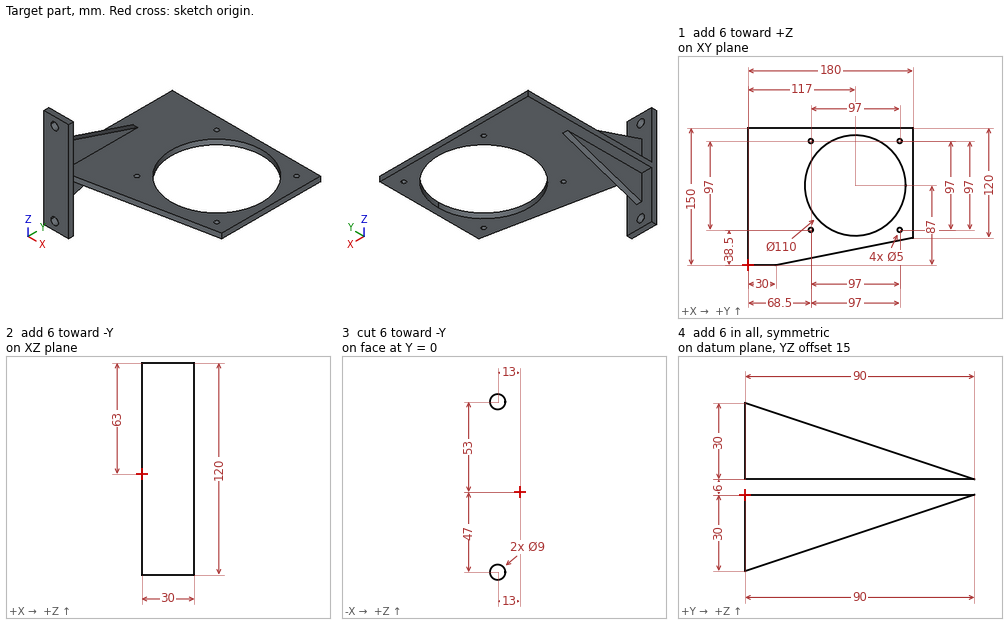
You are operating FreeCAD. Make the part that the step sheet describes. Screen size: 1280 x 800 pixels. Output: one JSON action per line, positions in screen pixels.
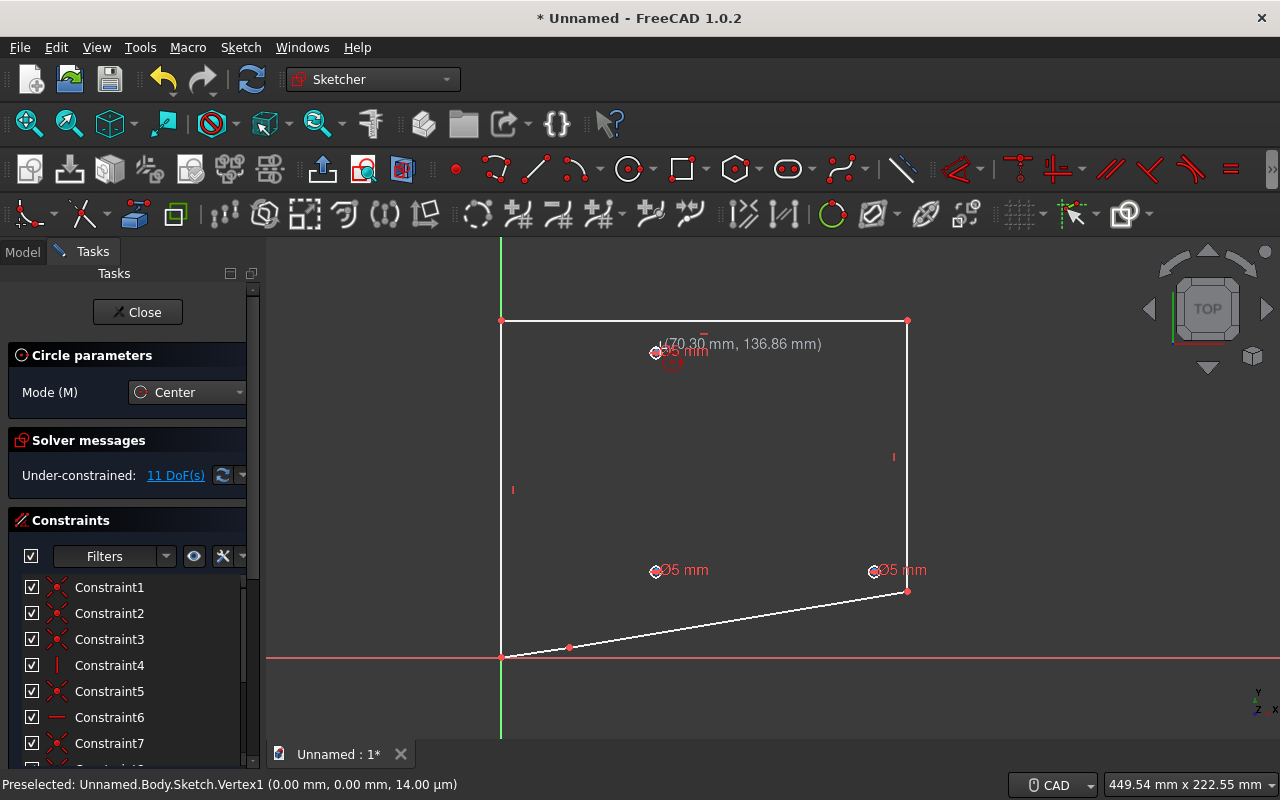
{"action": "left_click", "coordinate": [765, 461]}
{"action": "mouse_move", "coordinate": [853, 374]}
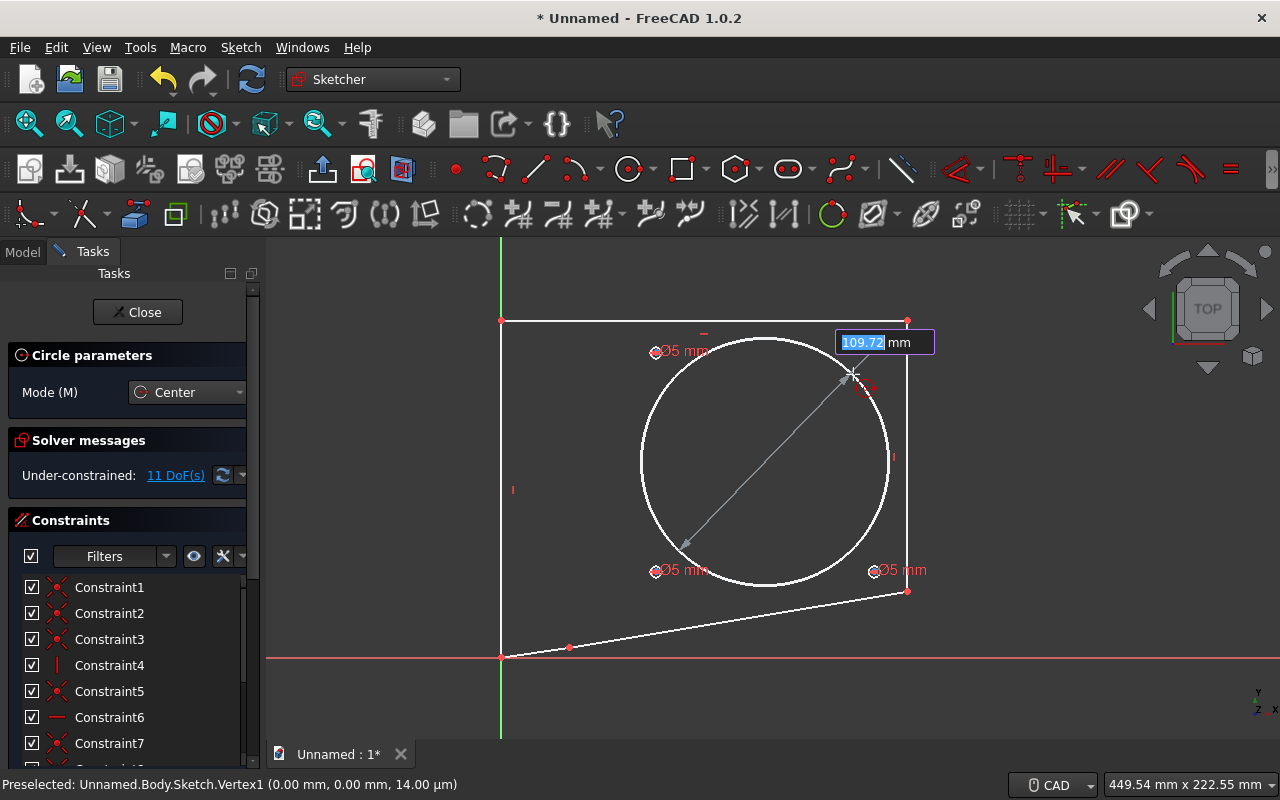
{"action": "type", "text": "110"}
{"action": "key", "text": "Return"}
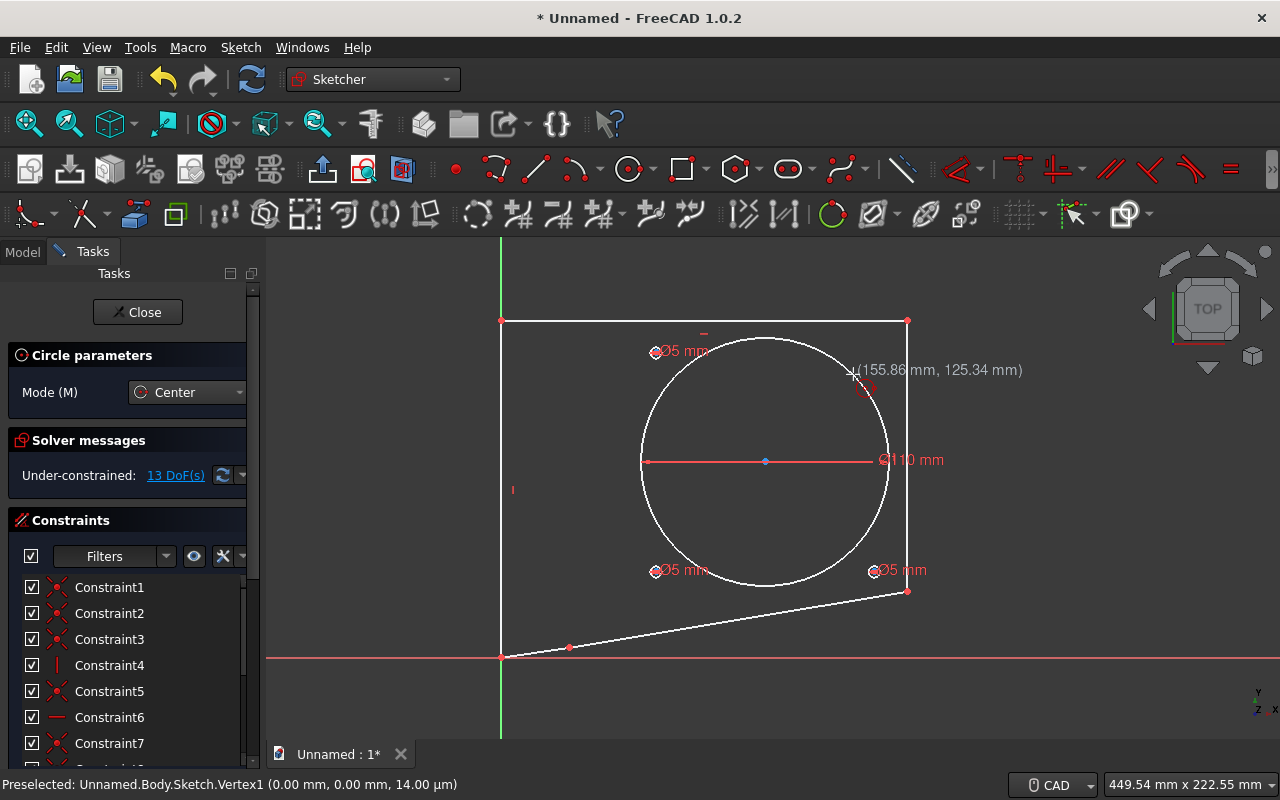
{"action": "scroll", "coordinate": [875, 352], "scroll_direction": "up", "scroll_amount": 7}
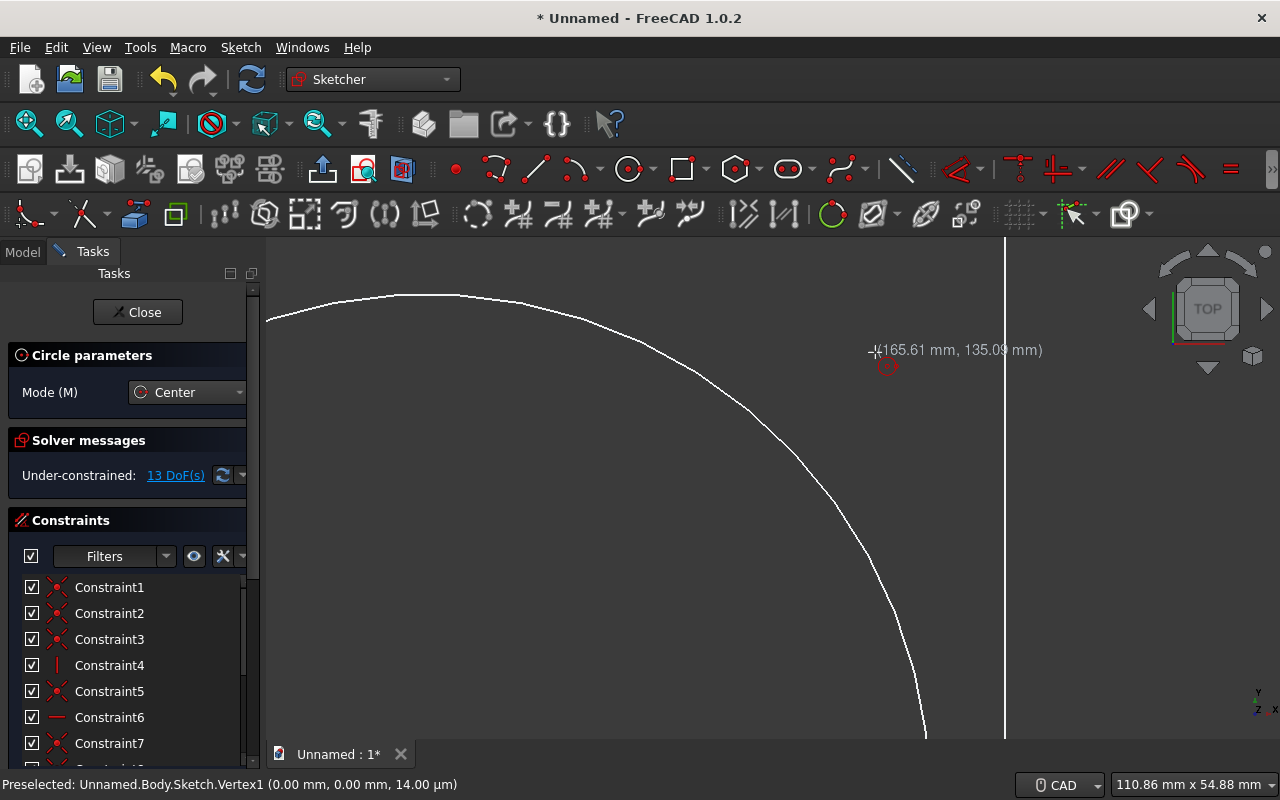
{"action": "scroll", "coordinate": [876, 352], "scroll_direction": "down", "scroll_amount": 7}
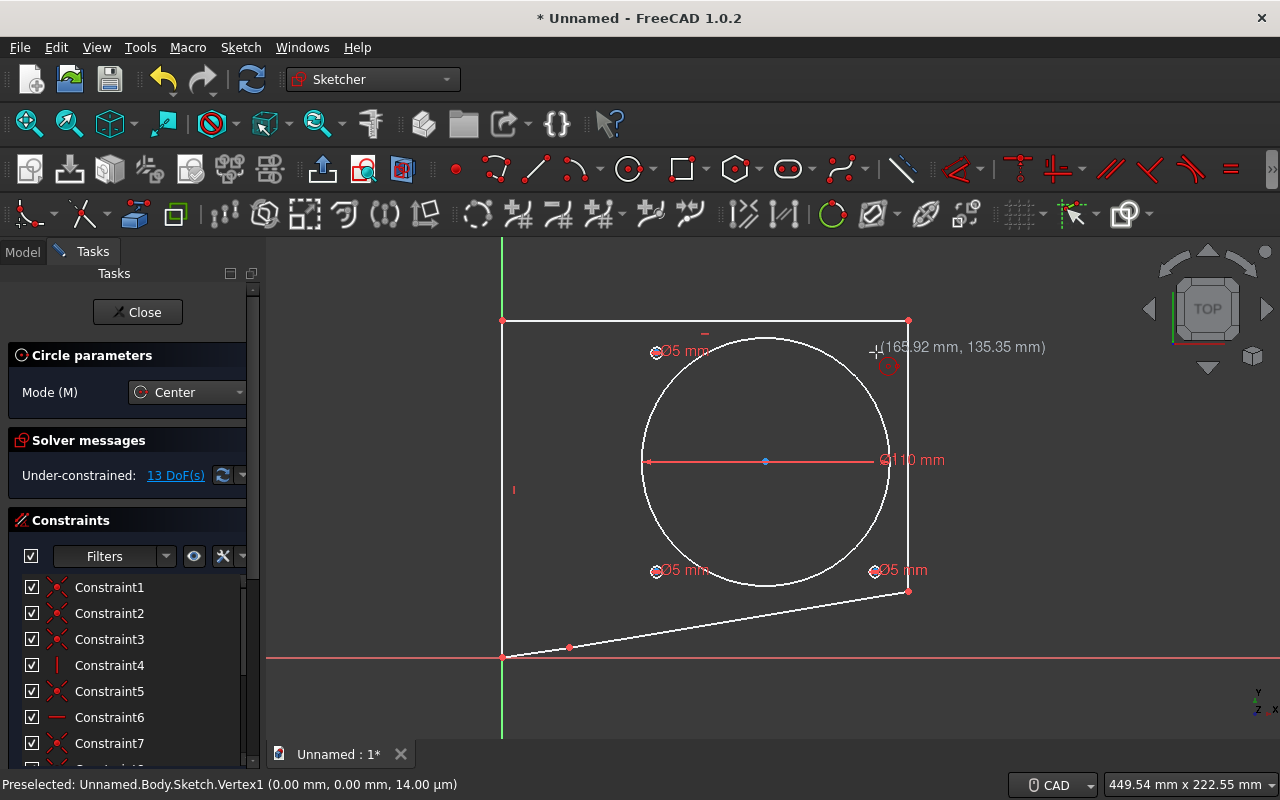
{"action": "left_click", "coordinate": [875, 352]}
{"action": "mouse_move", "coordinate": [879, 348]}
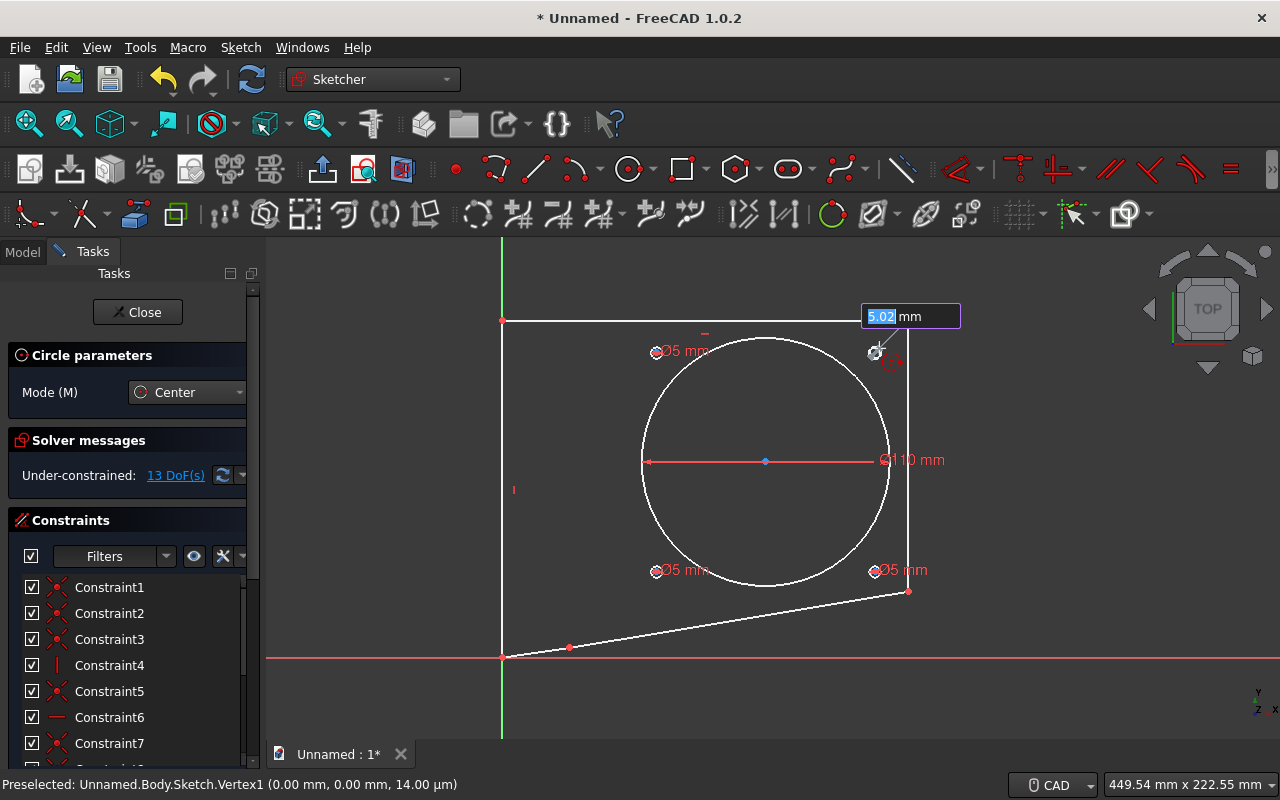
{"action": "type", "text": "5"}
{"action": "key", "text": "Return"}
{"action": "key", "text": "Escape"}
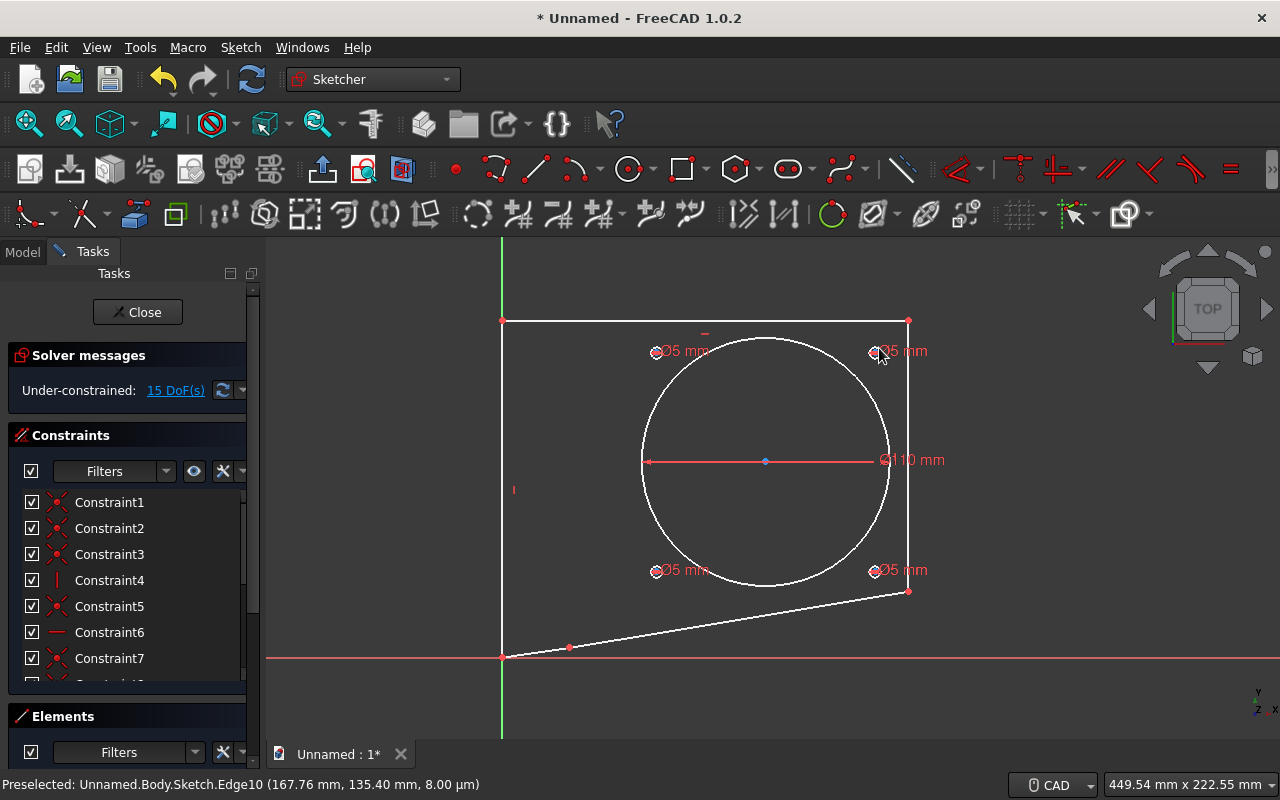
{"action": "left_click", "coordinate": [523, 655]}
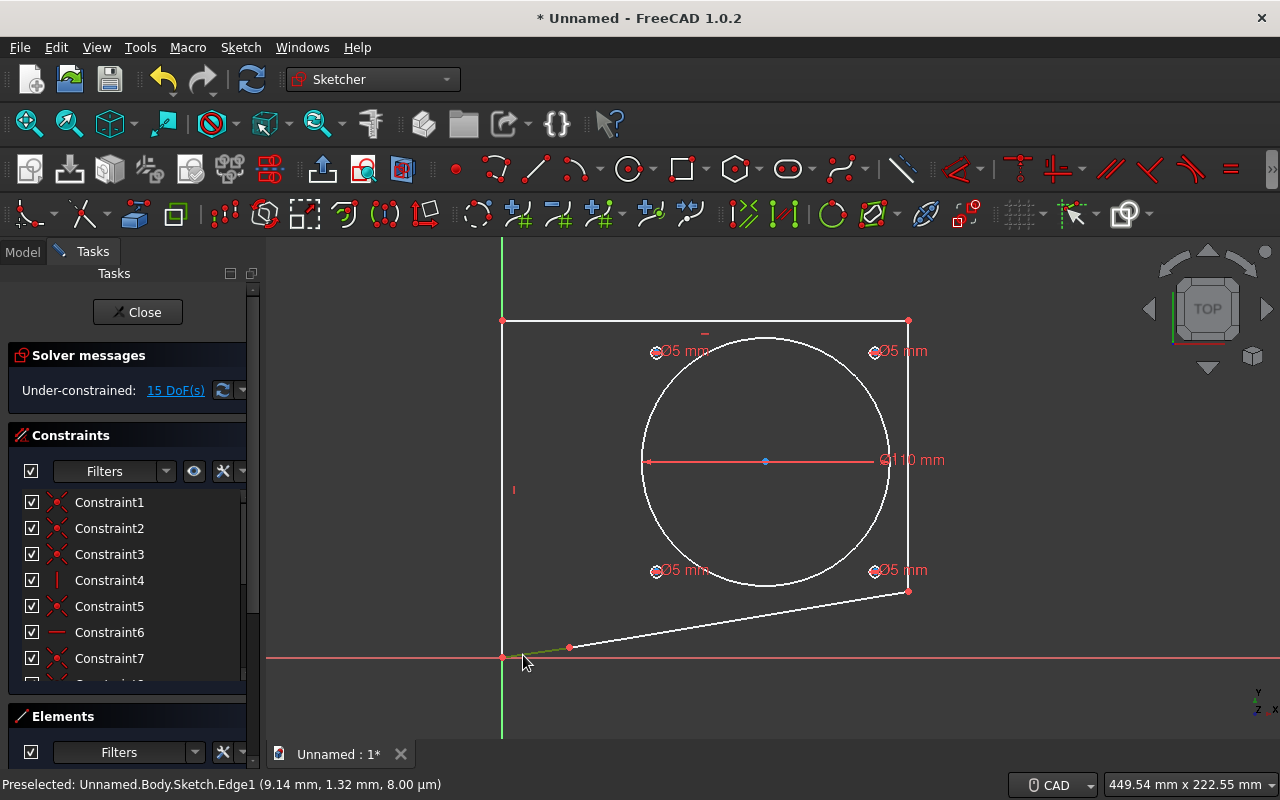
{"action": "key", "text": "h"}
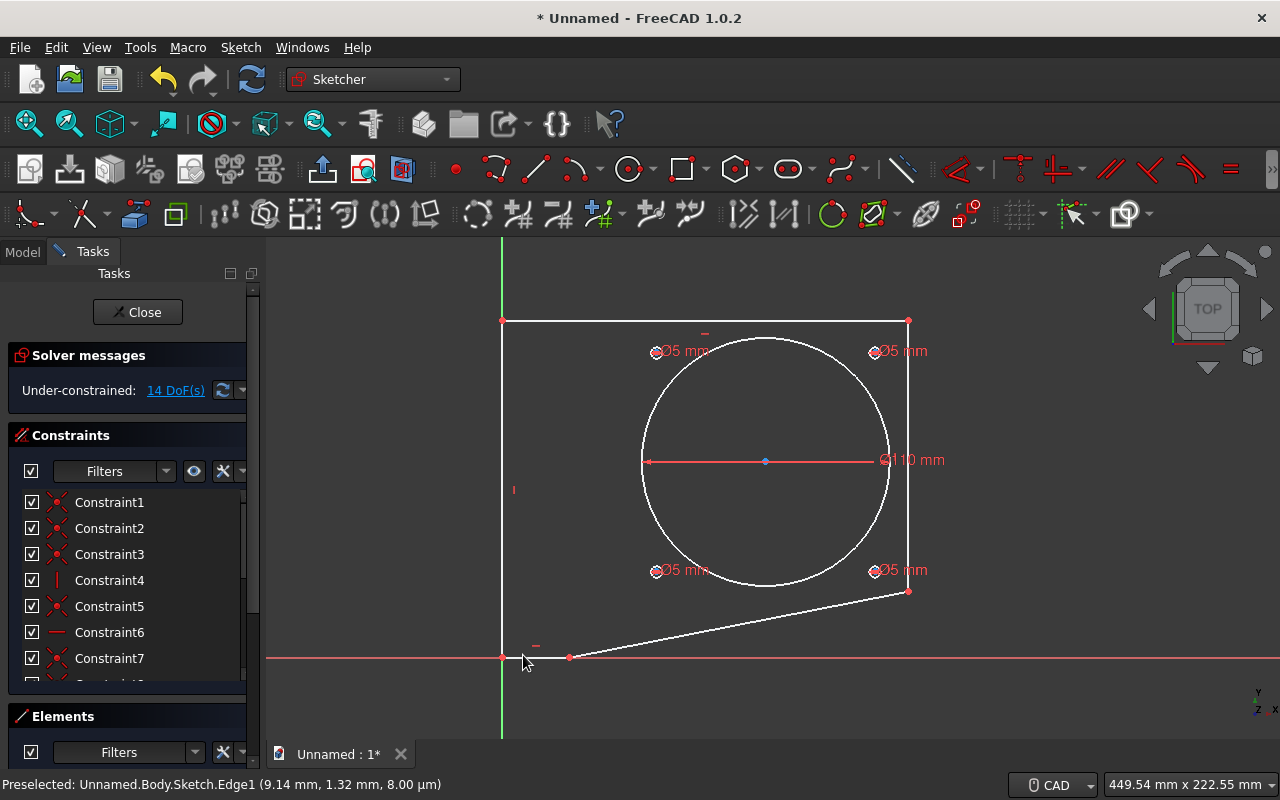
{"action": "left_click", "coordinate": [523, 658]}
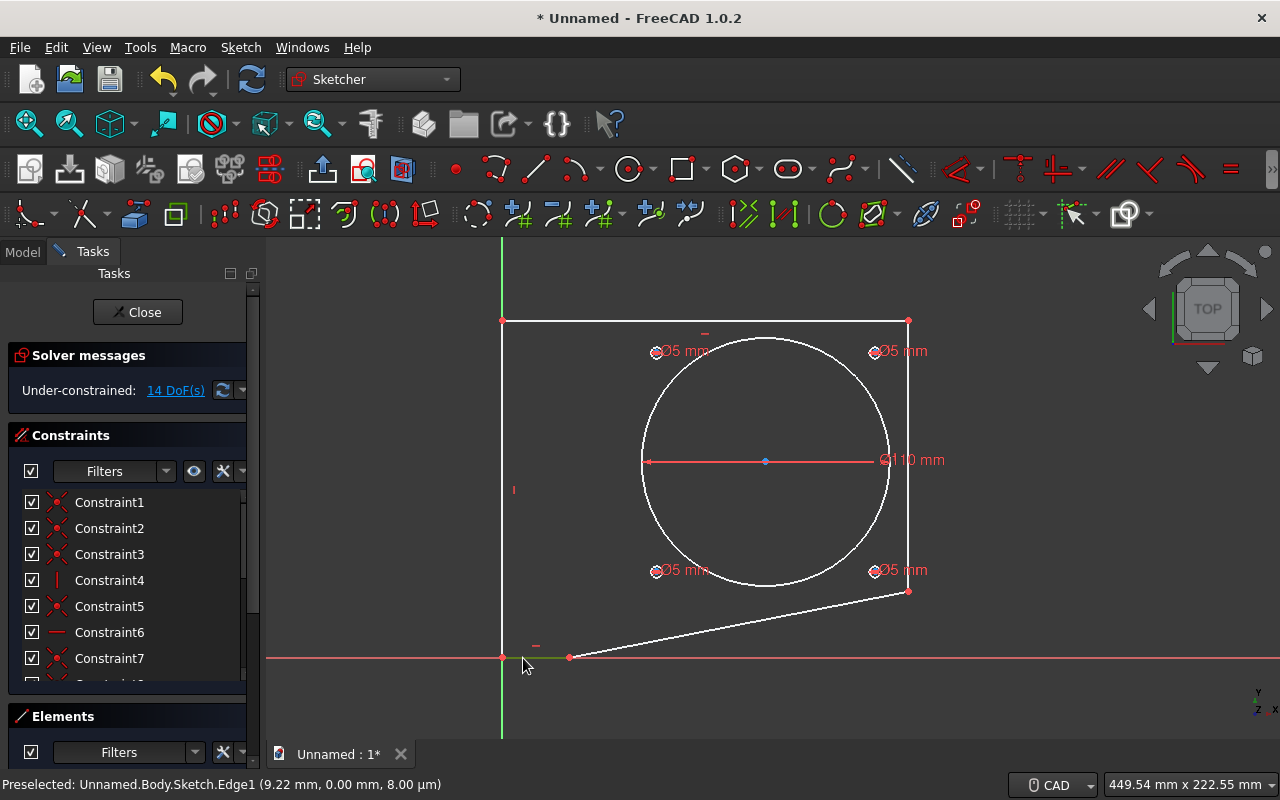
{"action": "left_click", "coordinate": [982, 170]}